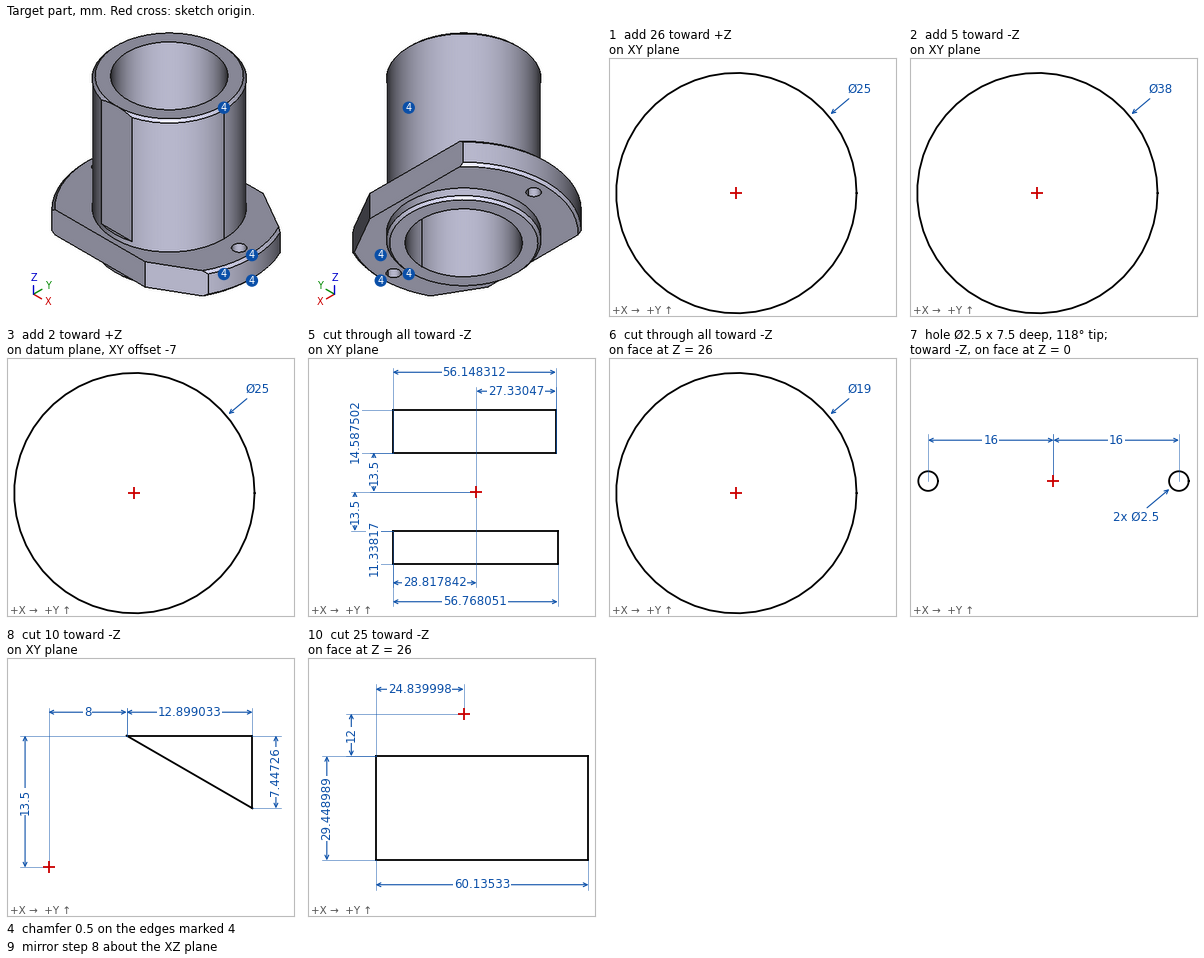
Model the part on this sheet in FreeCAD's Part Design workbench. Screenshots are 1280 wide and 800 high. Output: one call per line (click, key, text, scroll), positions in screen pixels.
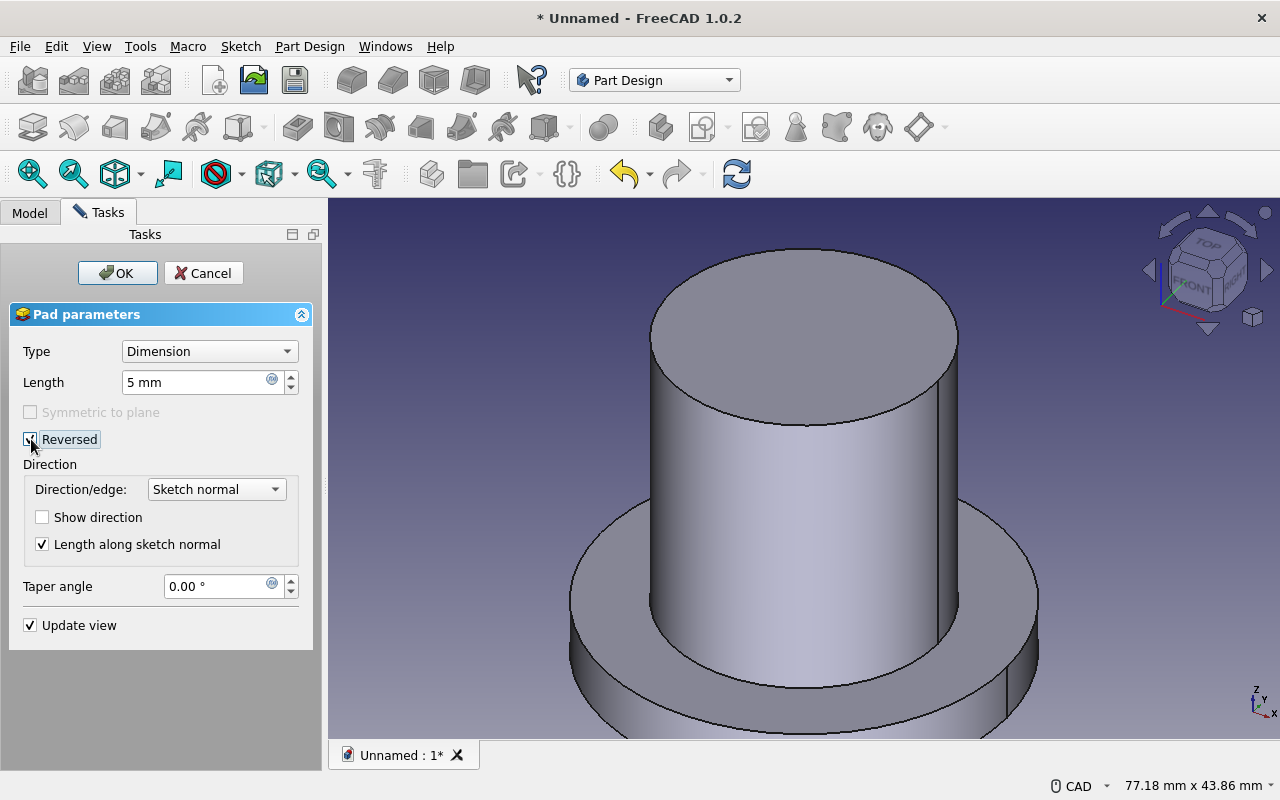
click(118, 273)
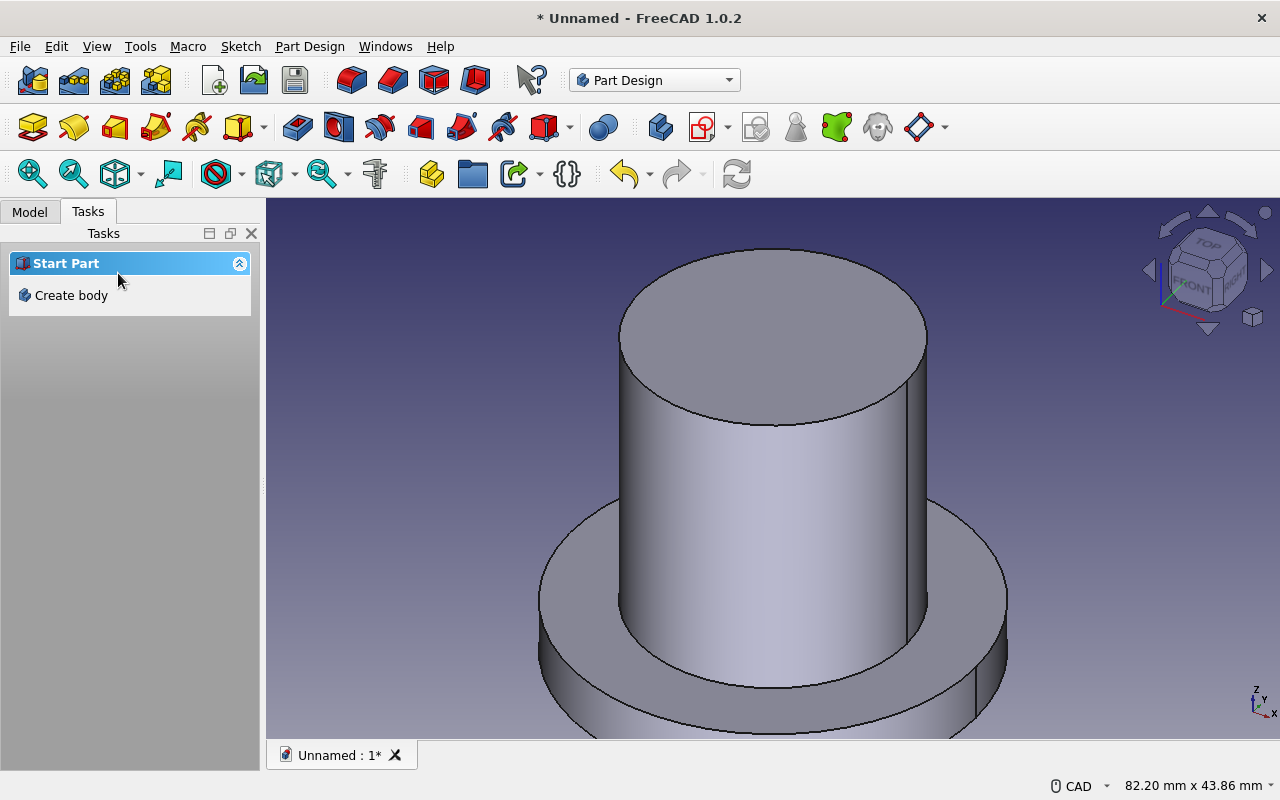
click(33, 174)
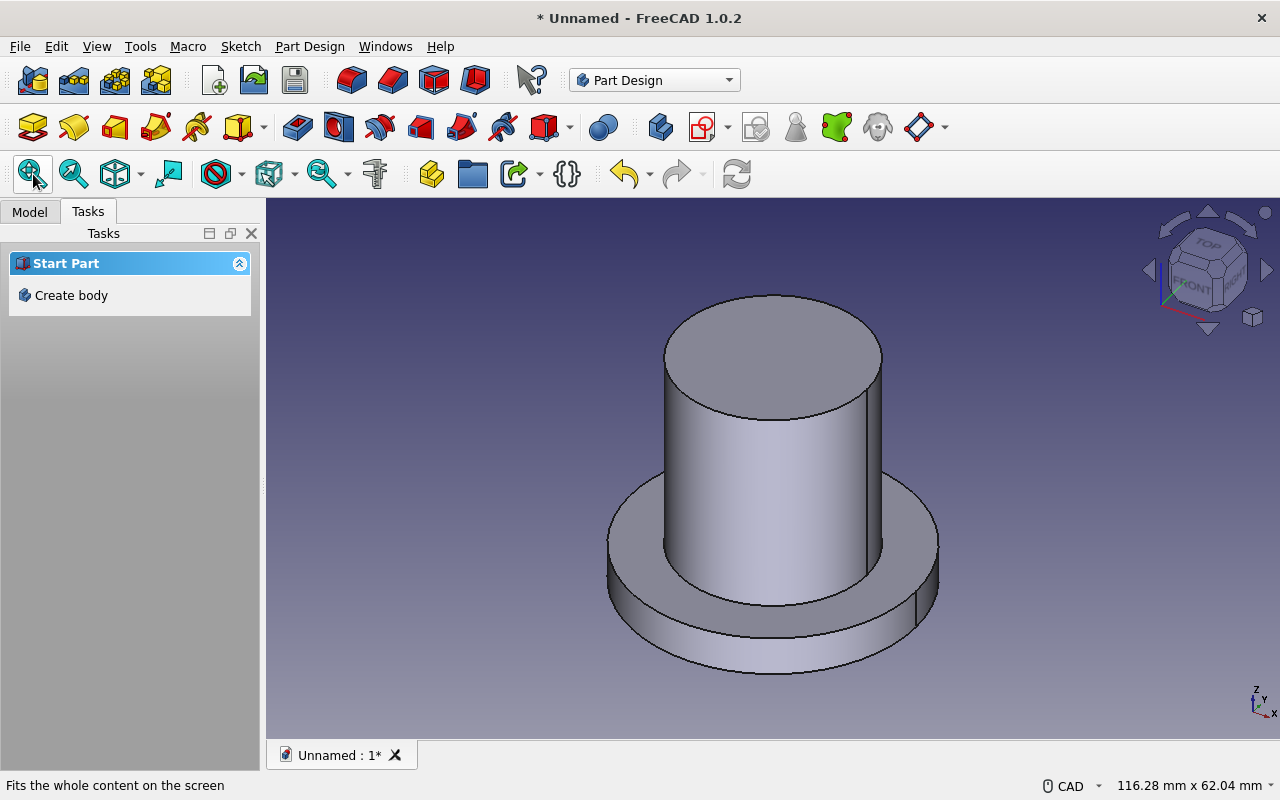
click(30, 212)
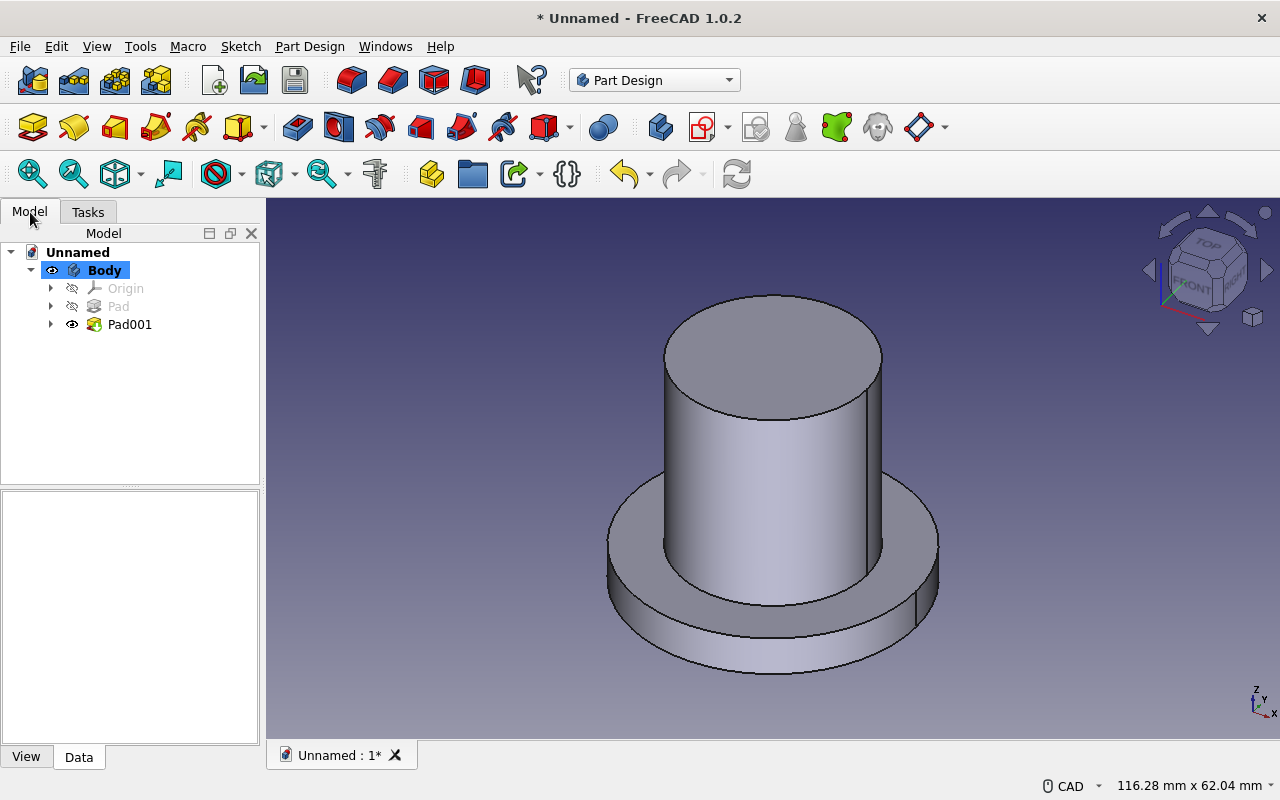
click(51, 288)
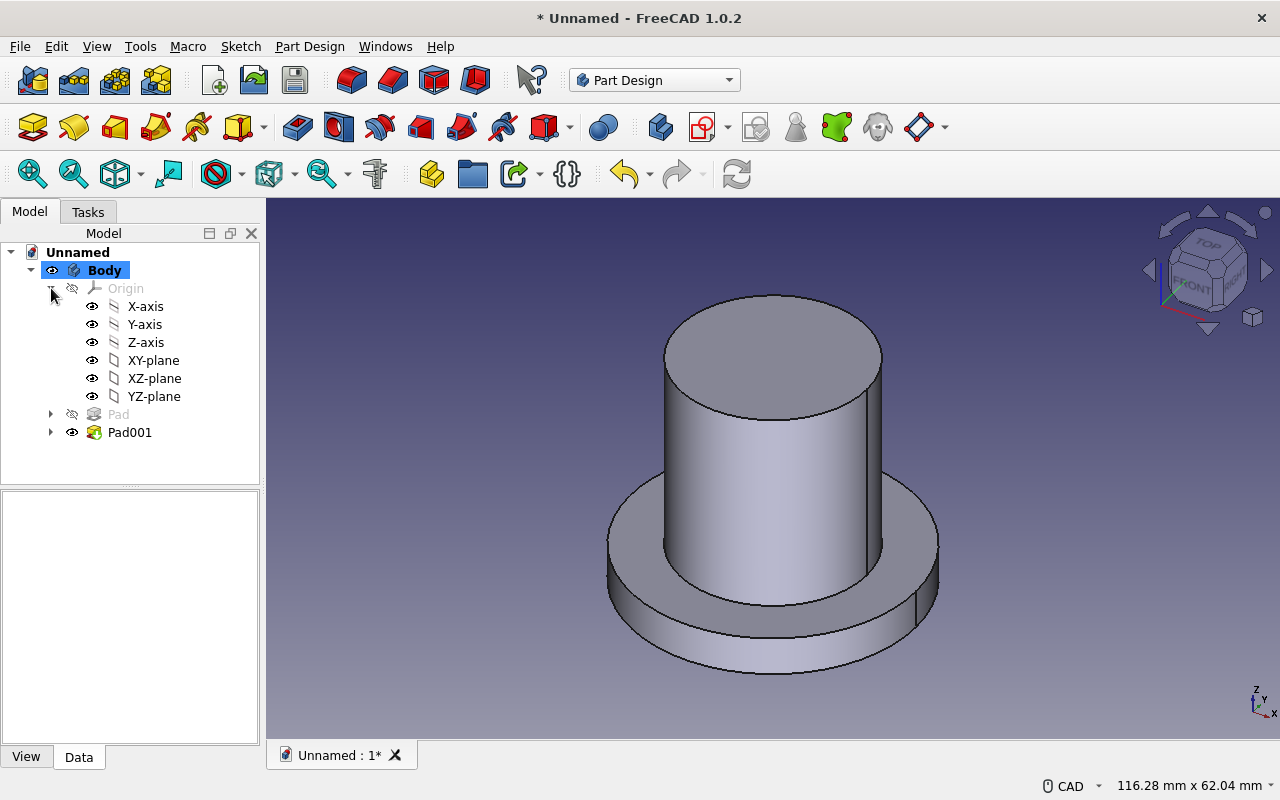
click(137, 360)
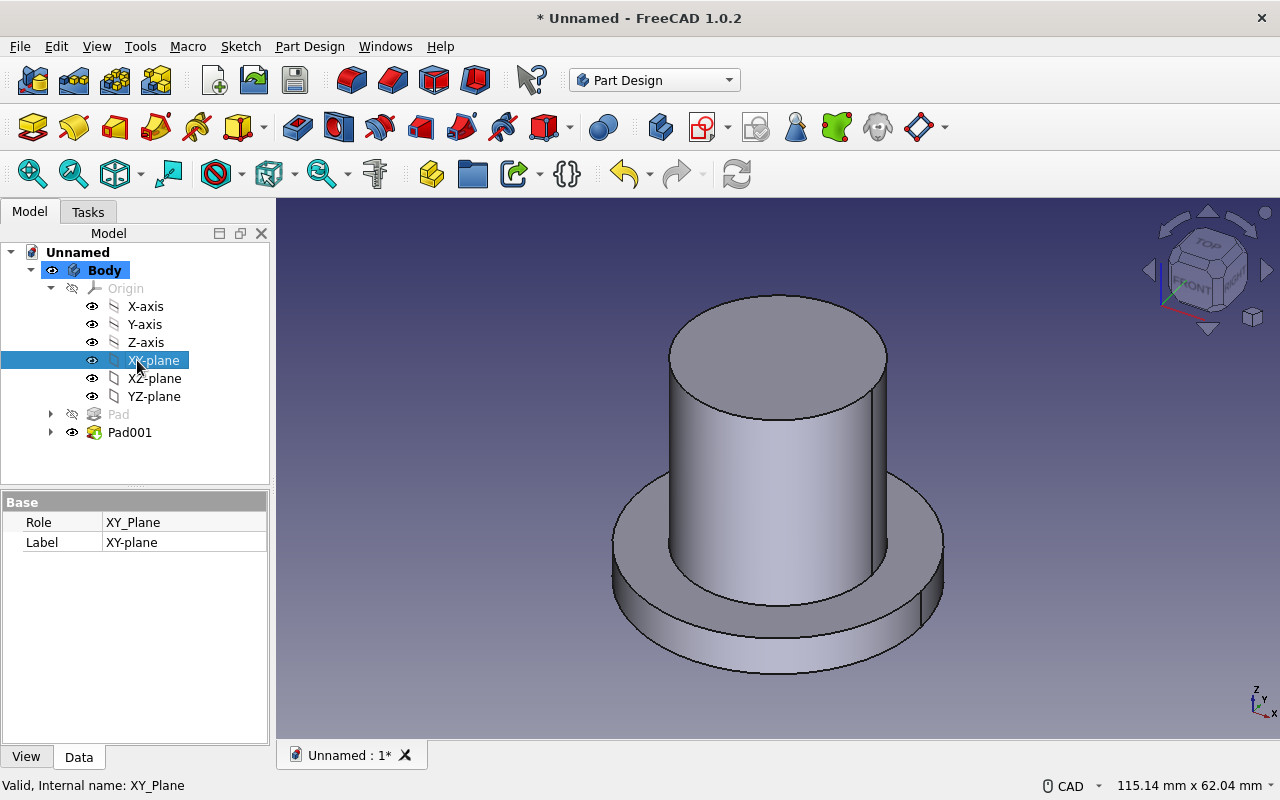
click(918, 128)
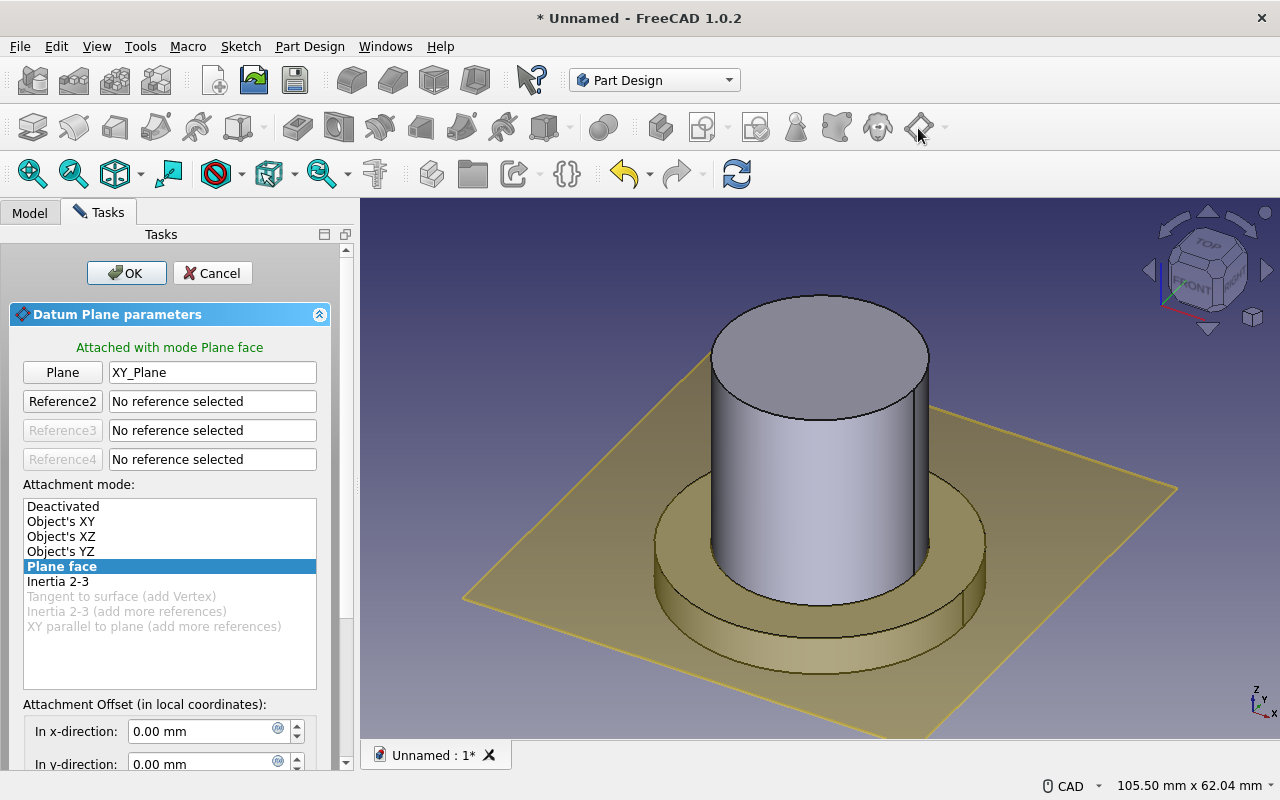
scroll(346, 507, down, 2)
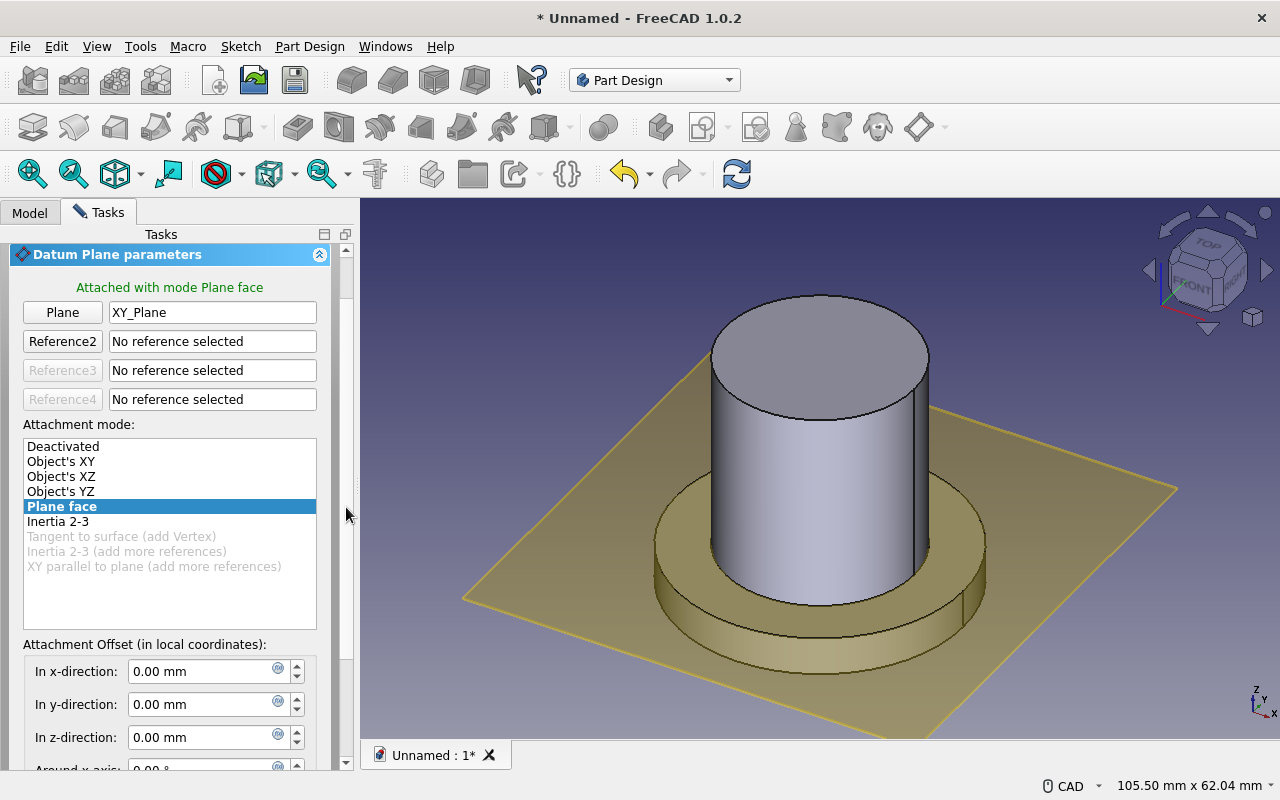
triple_click(210, 678)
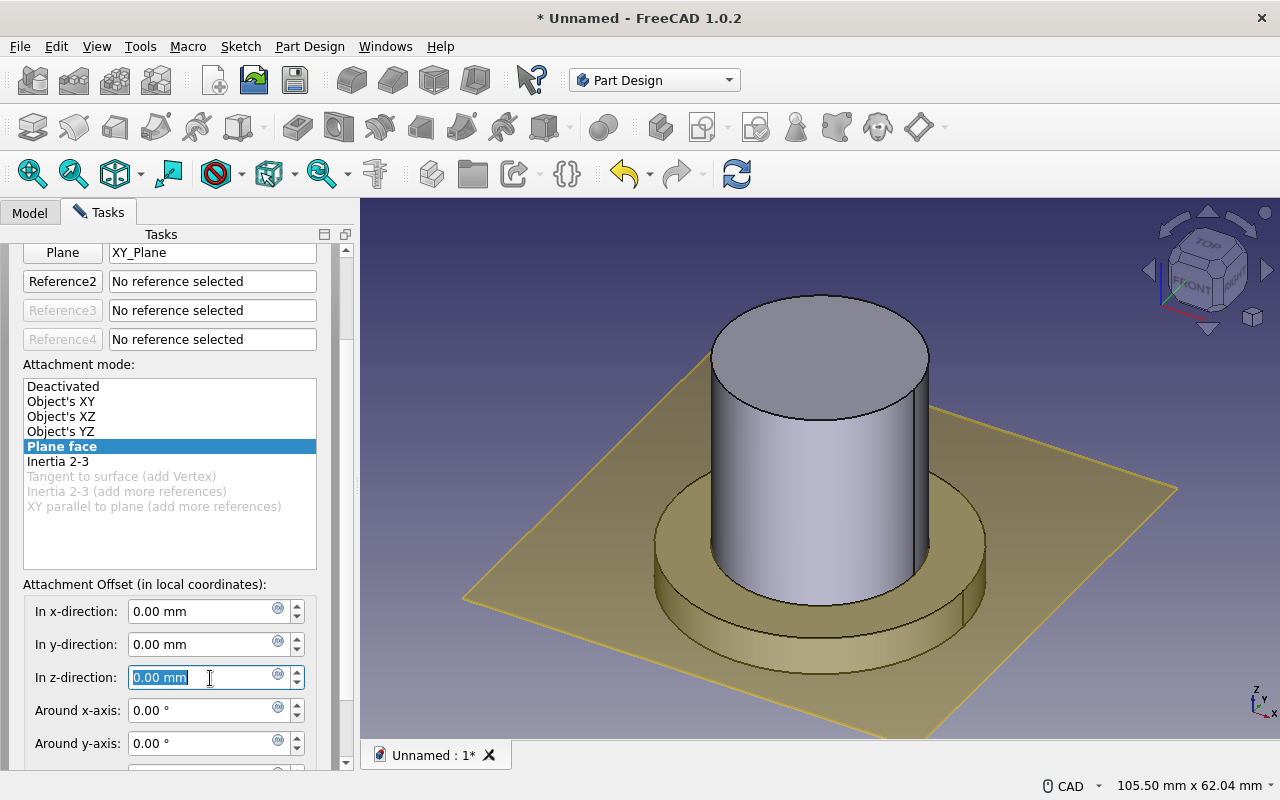
text(-7)
key(Tab)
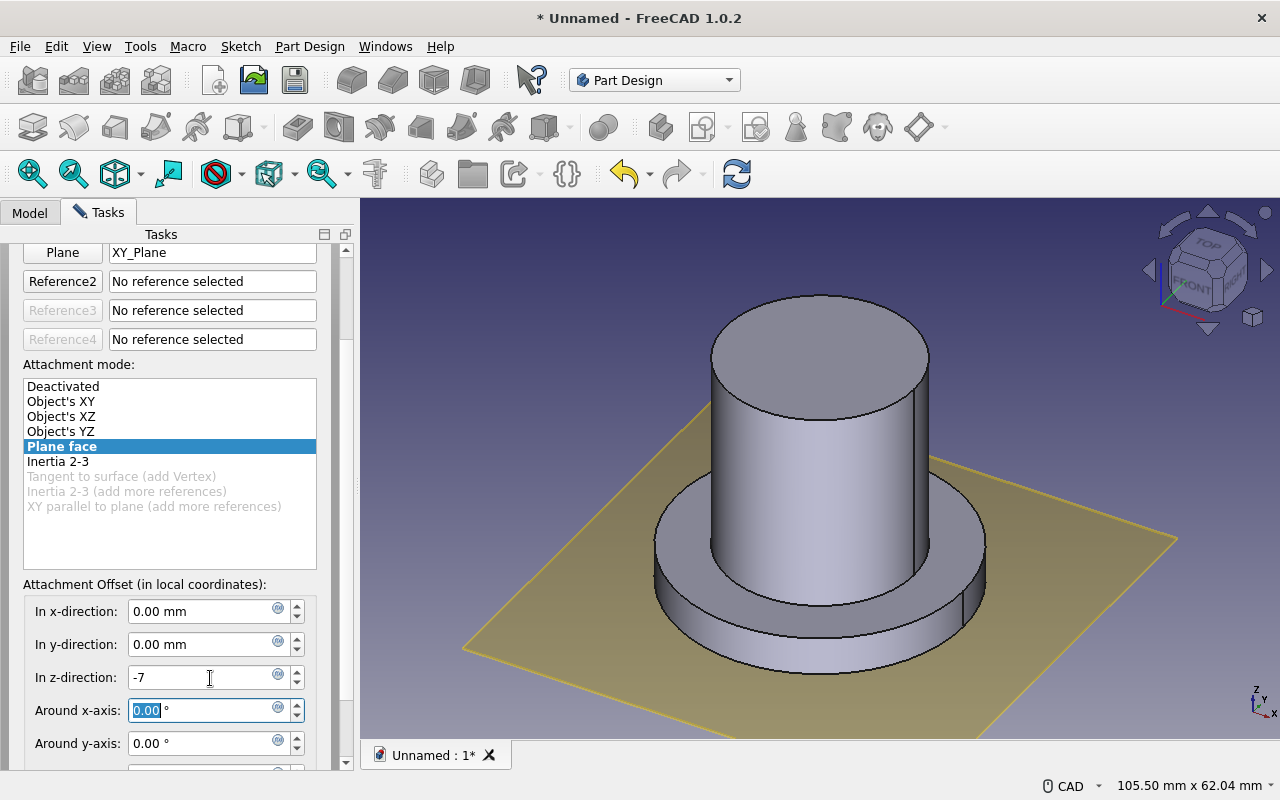
scroll(346, 507, up, 3)